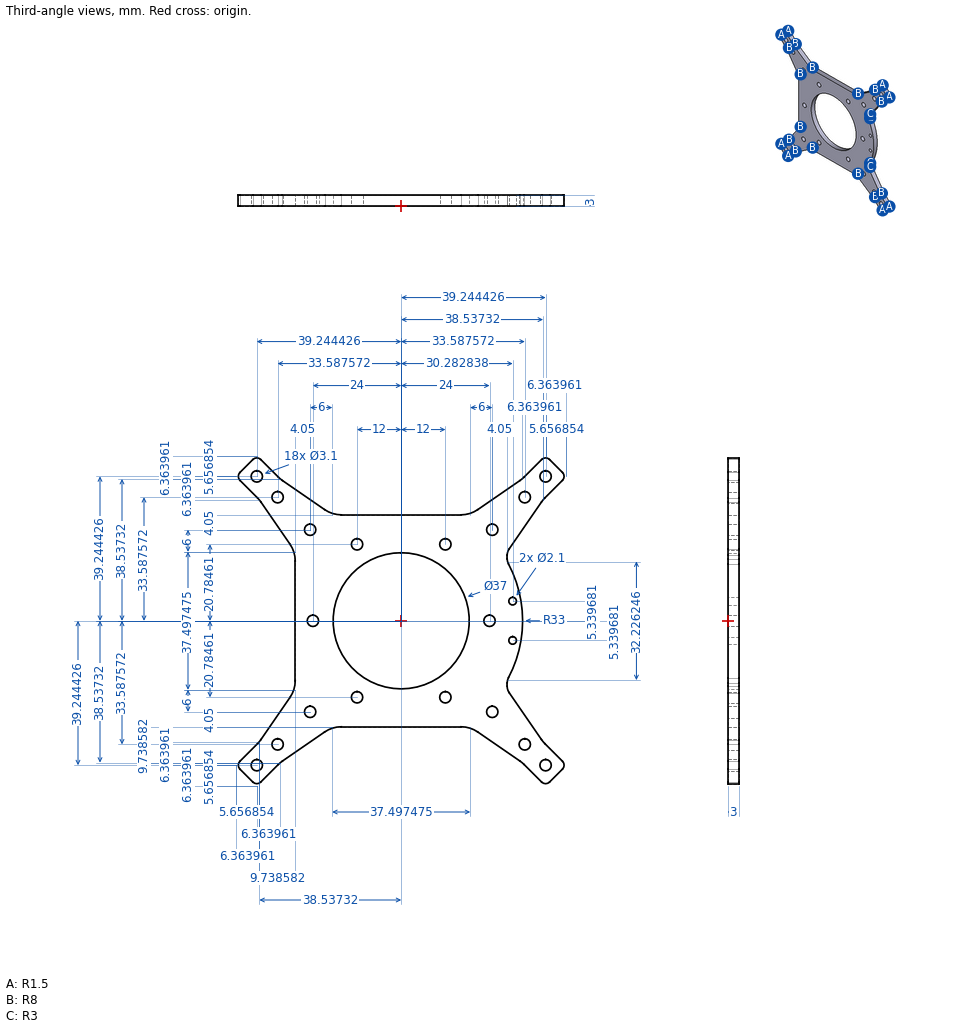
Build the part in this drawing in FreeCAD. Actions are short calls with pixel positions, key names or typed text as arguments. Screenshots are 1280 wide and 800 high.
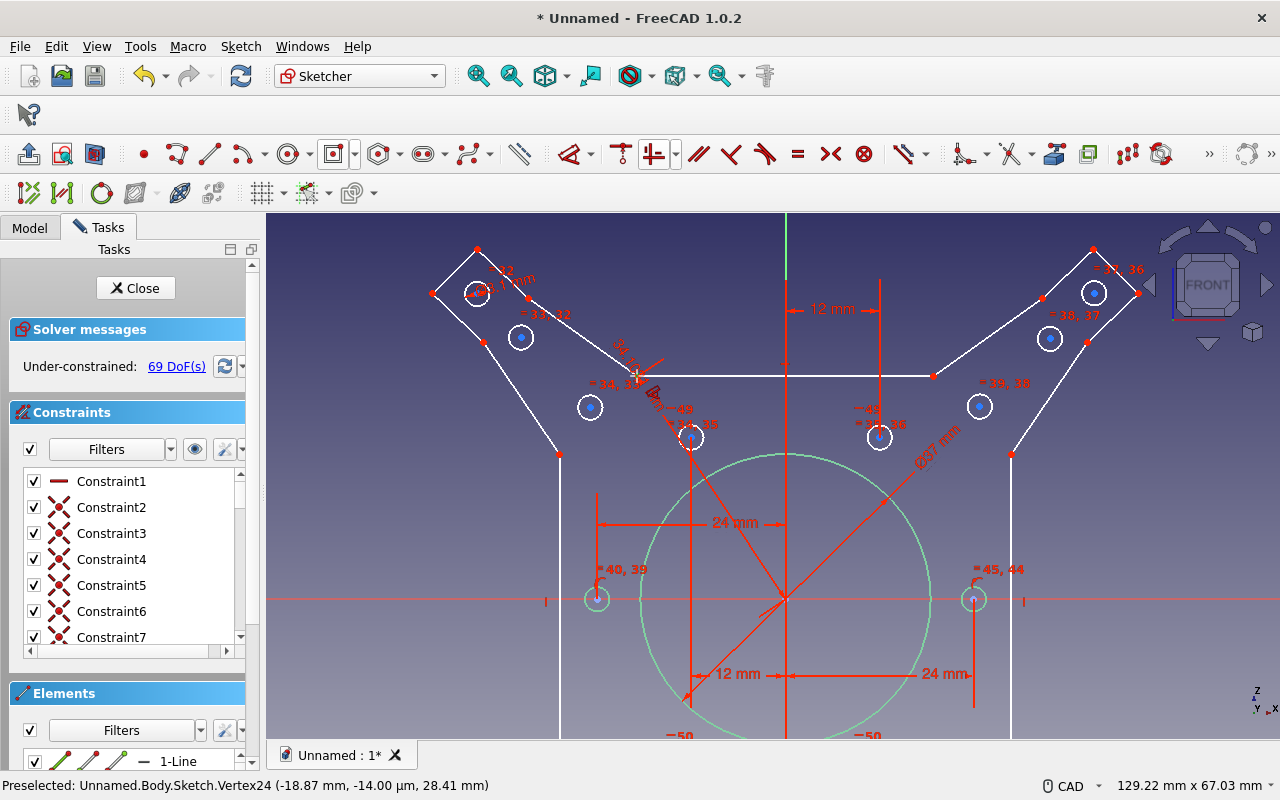
click(590, 408)
click(614, 342)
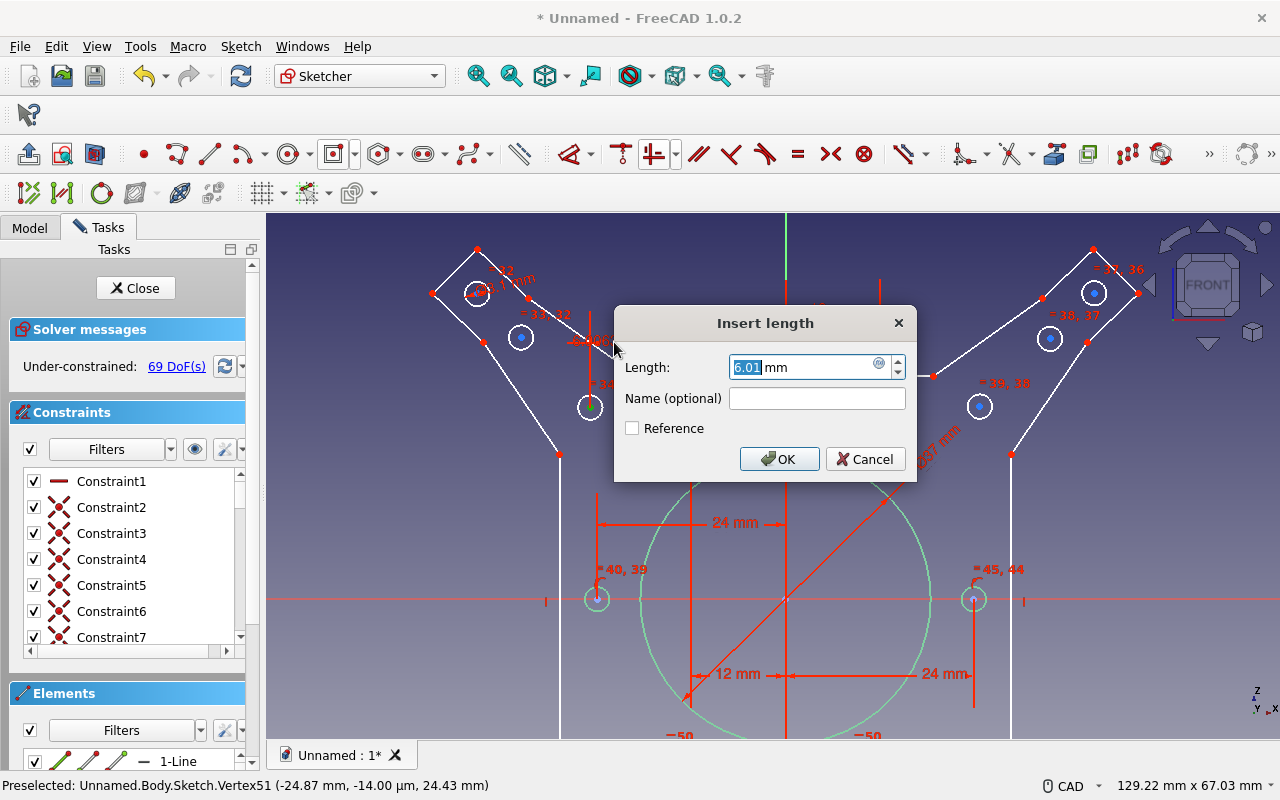
text(6)
key(Return)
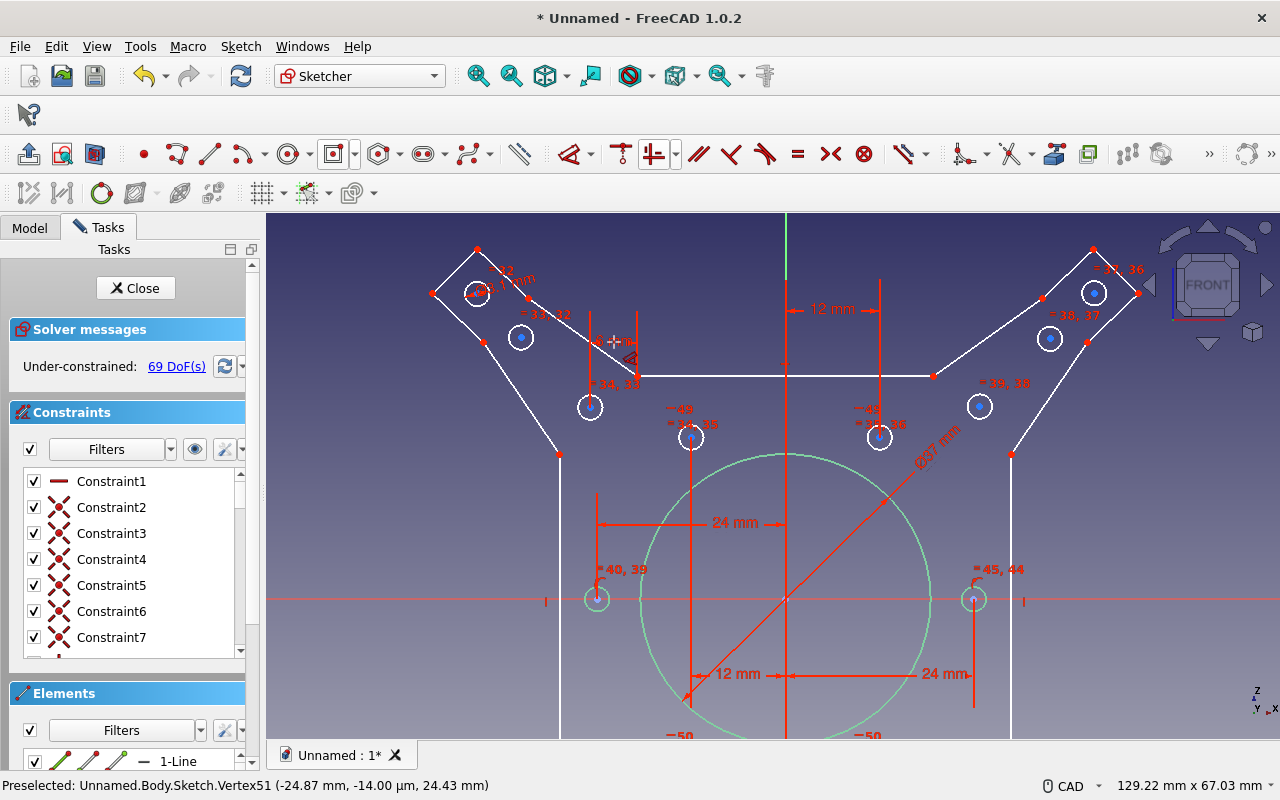
click(560, 454)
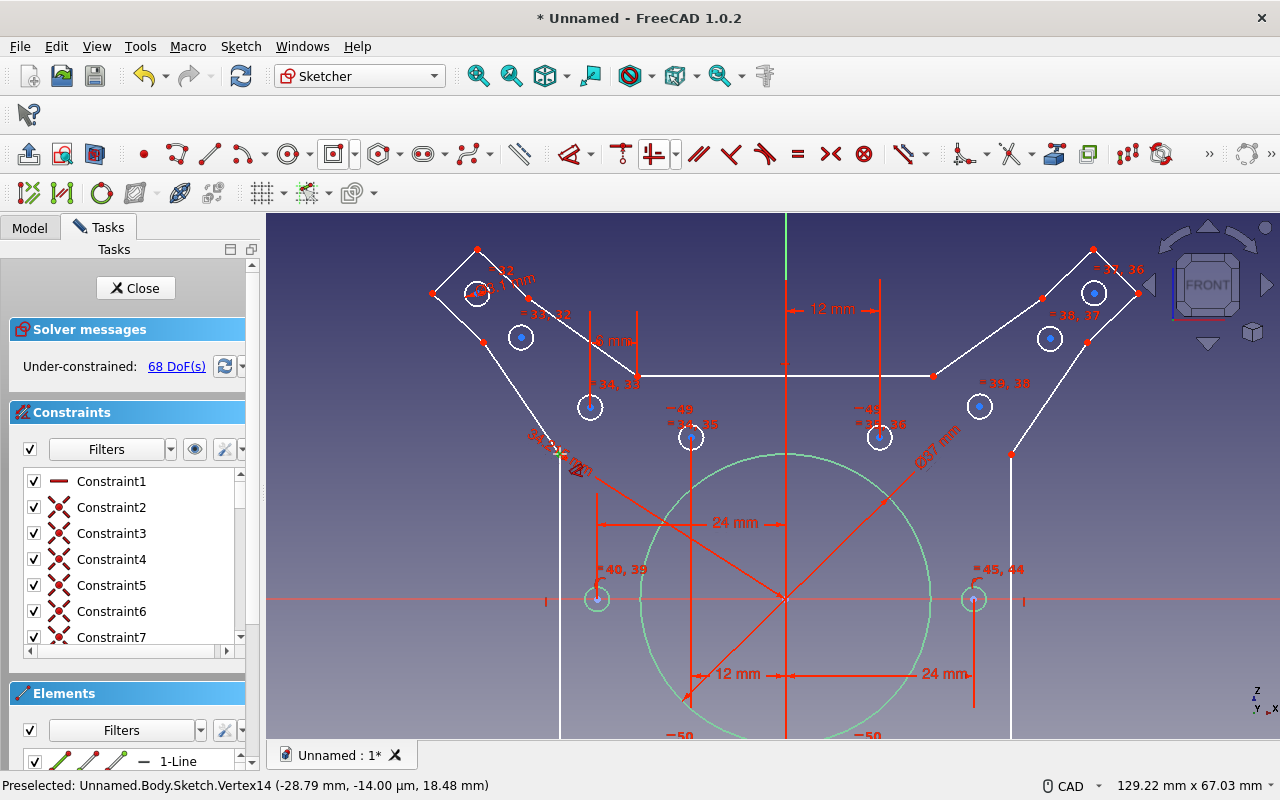
click(590, 408)
click(526, 431)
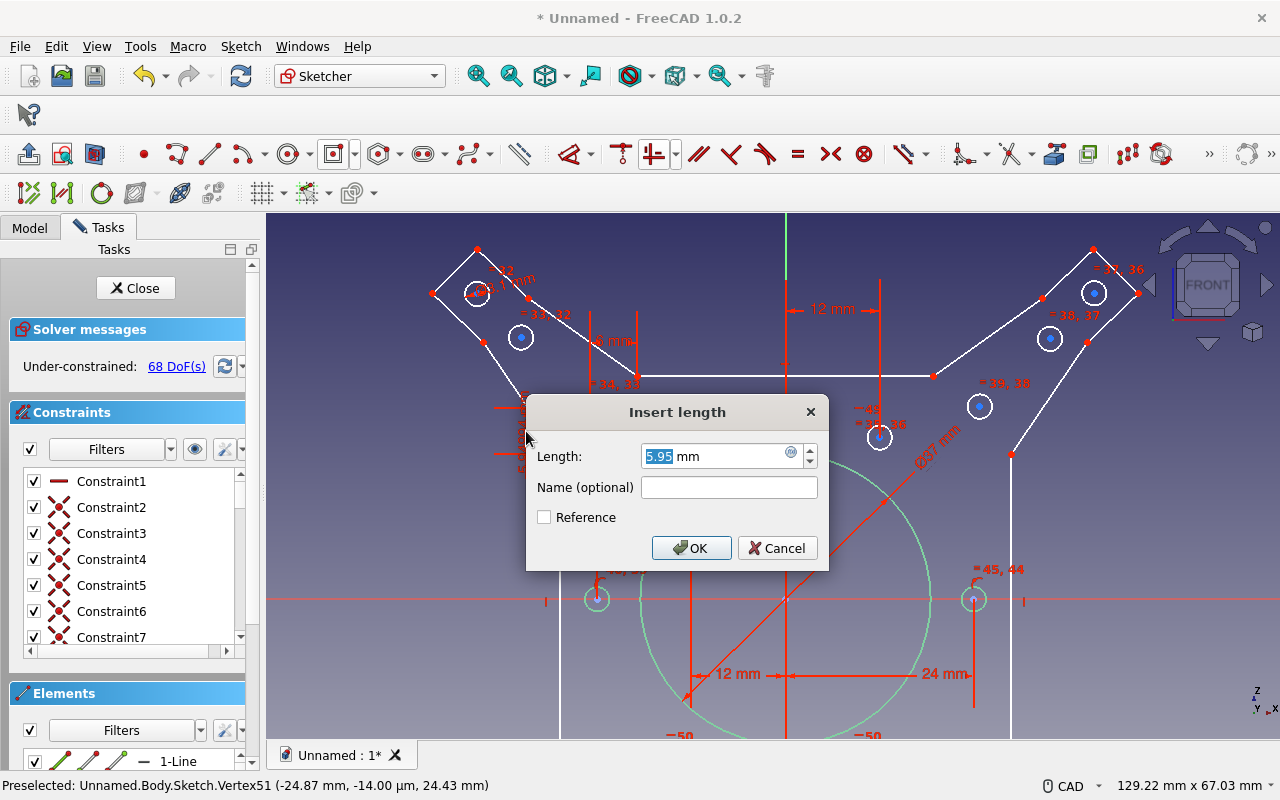
text(6)
key(Return)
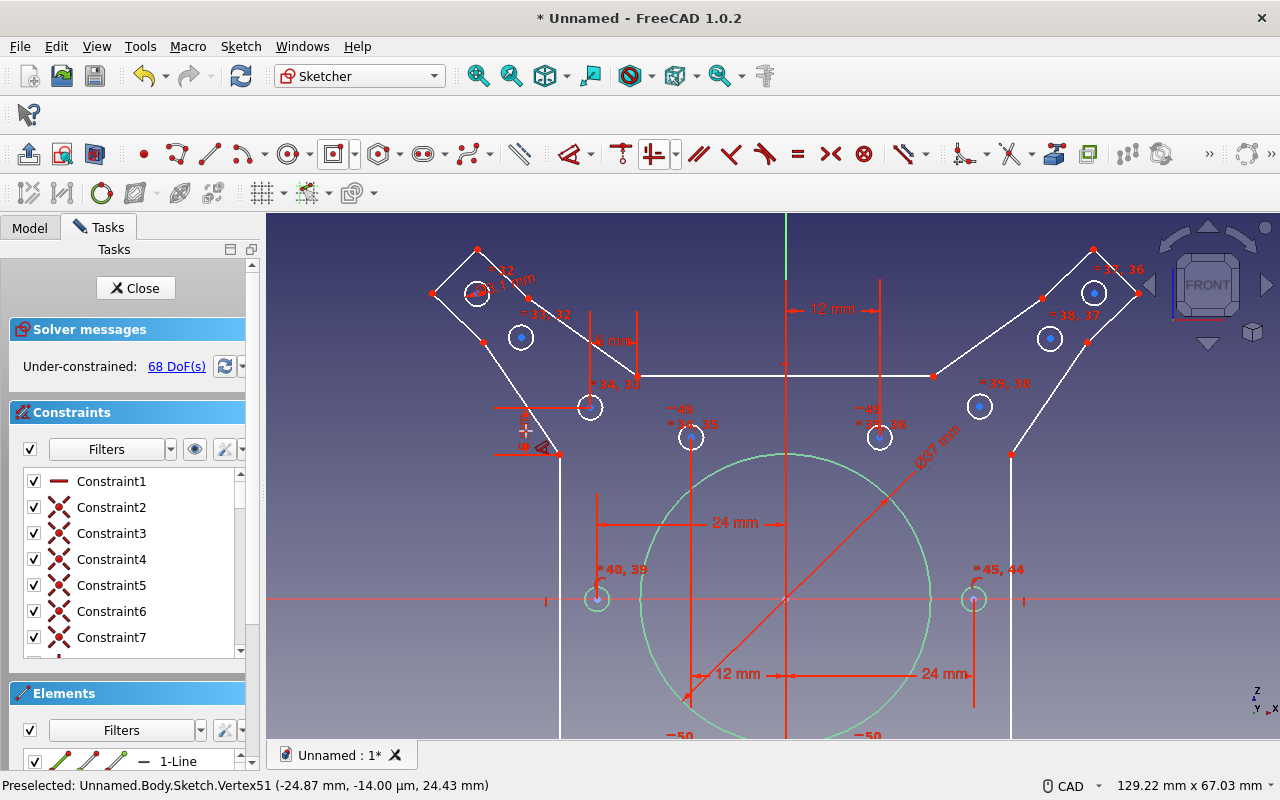
click(933, 376)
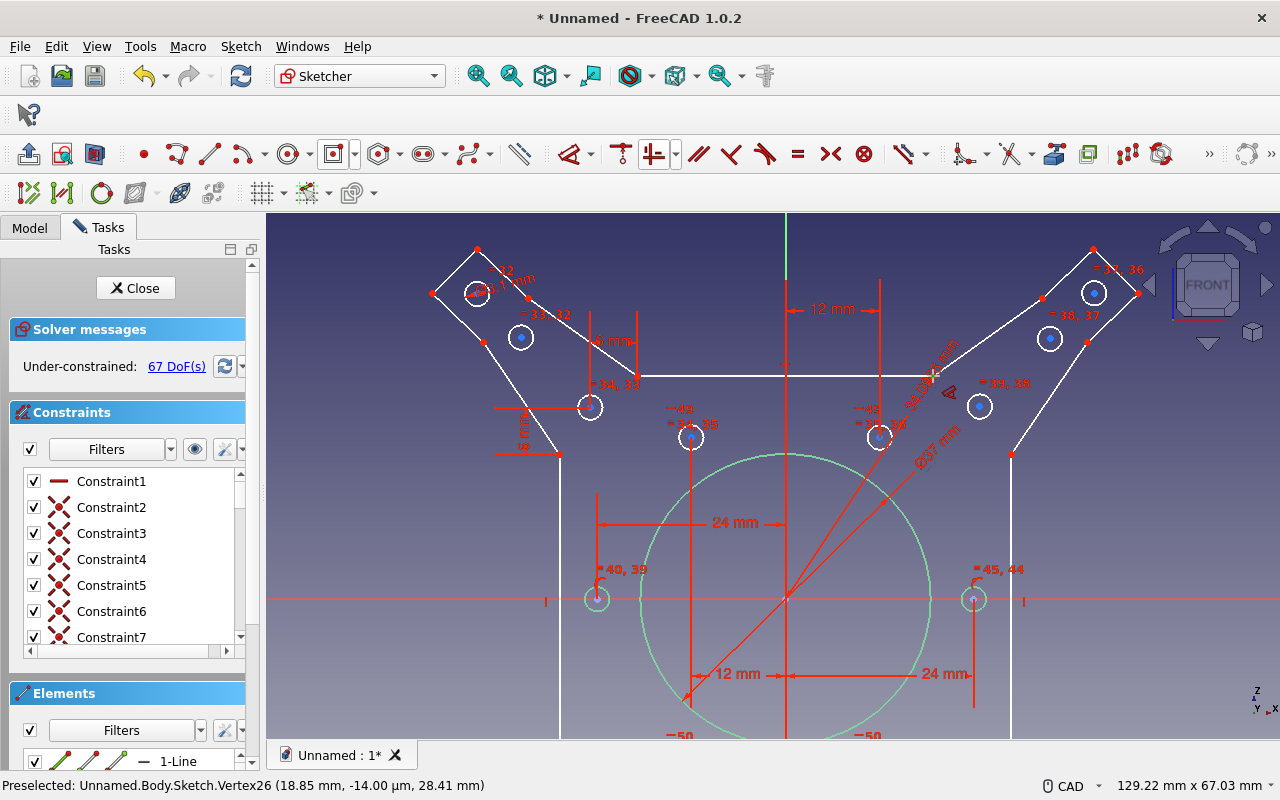
click(980, 407)
click(957, 342)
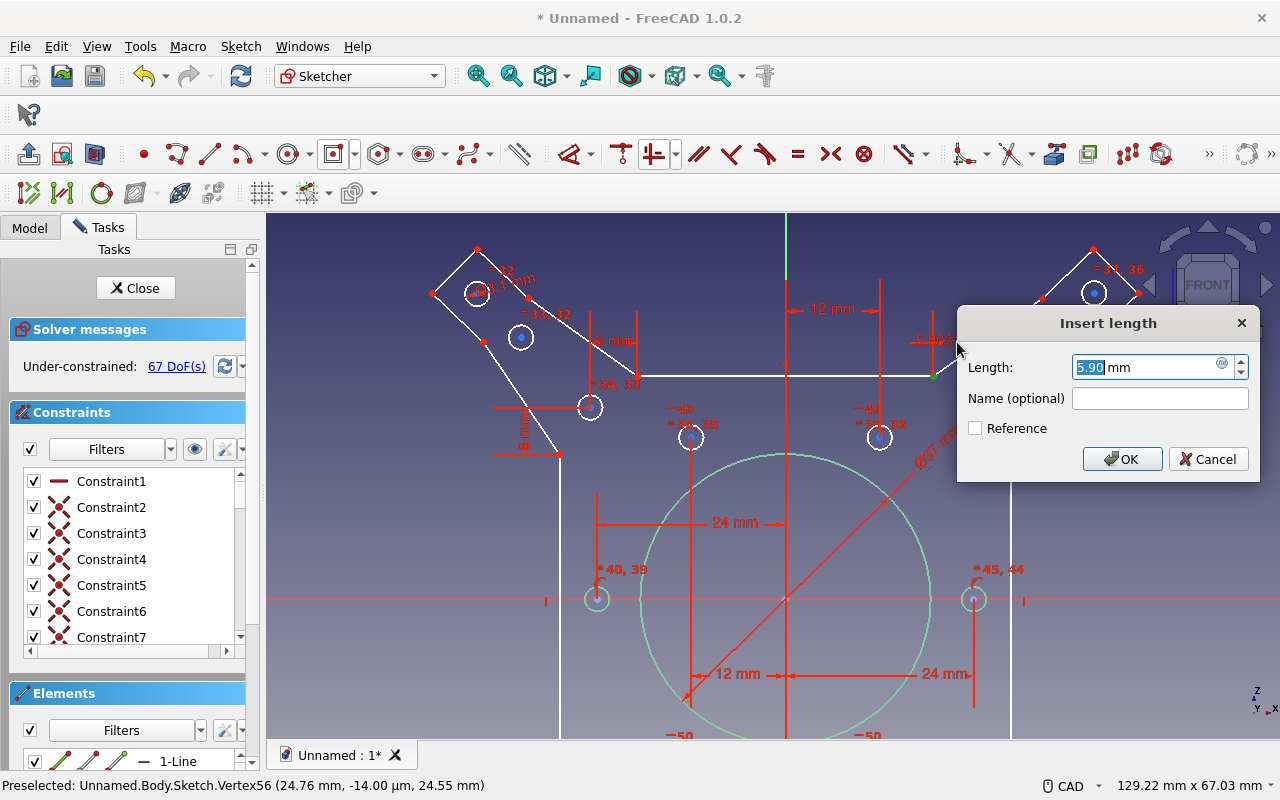
text(6)
key(Return)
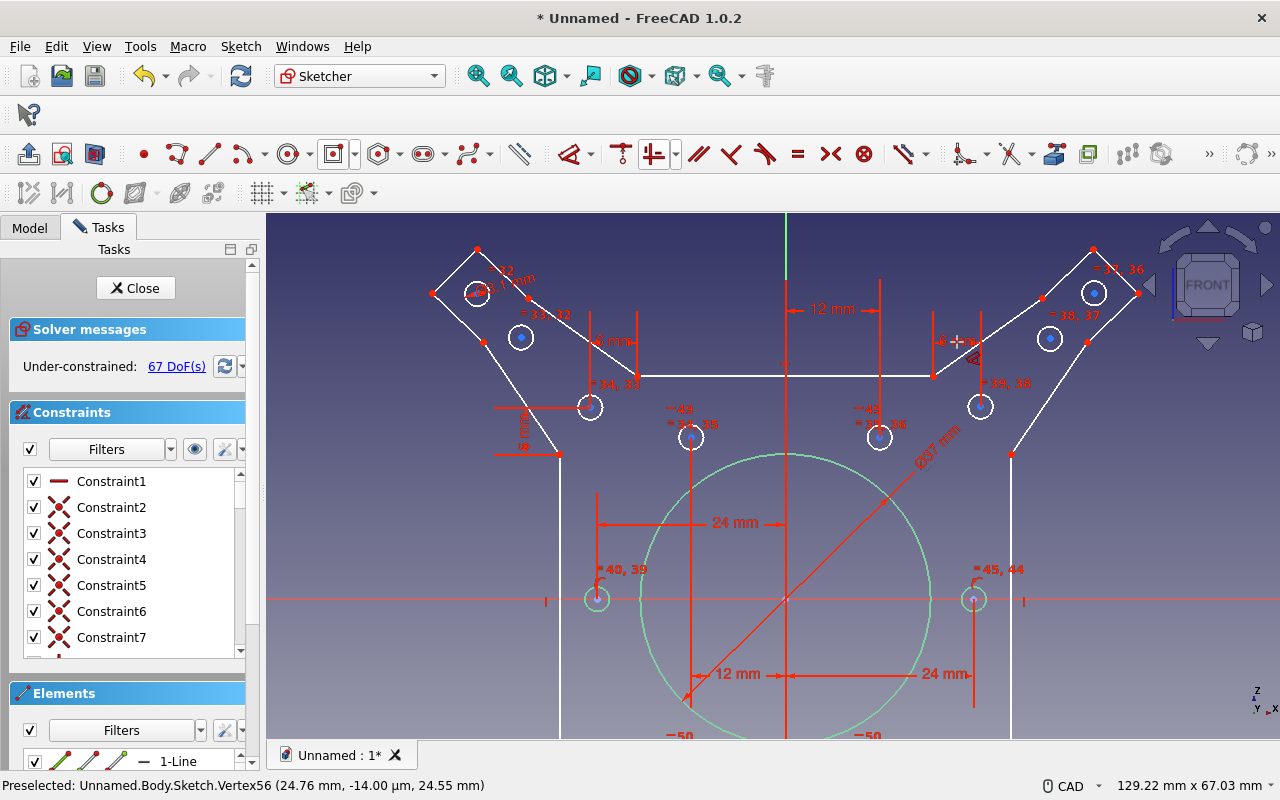
click(1011, 454)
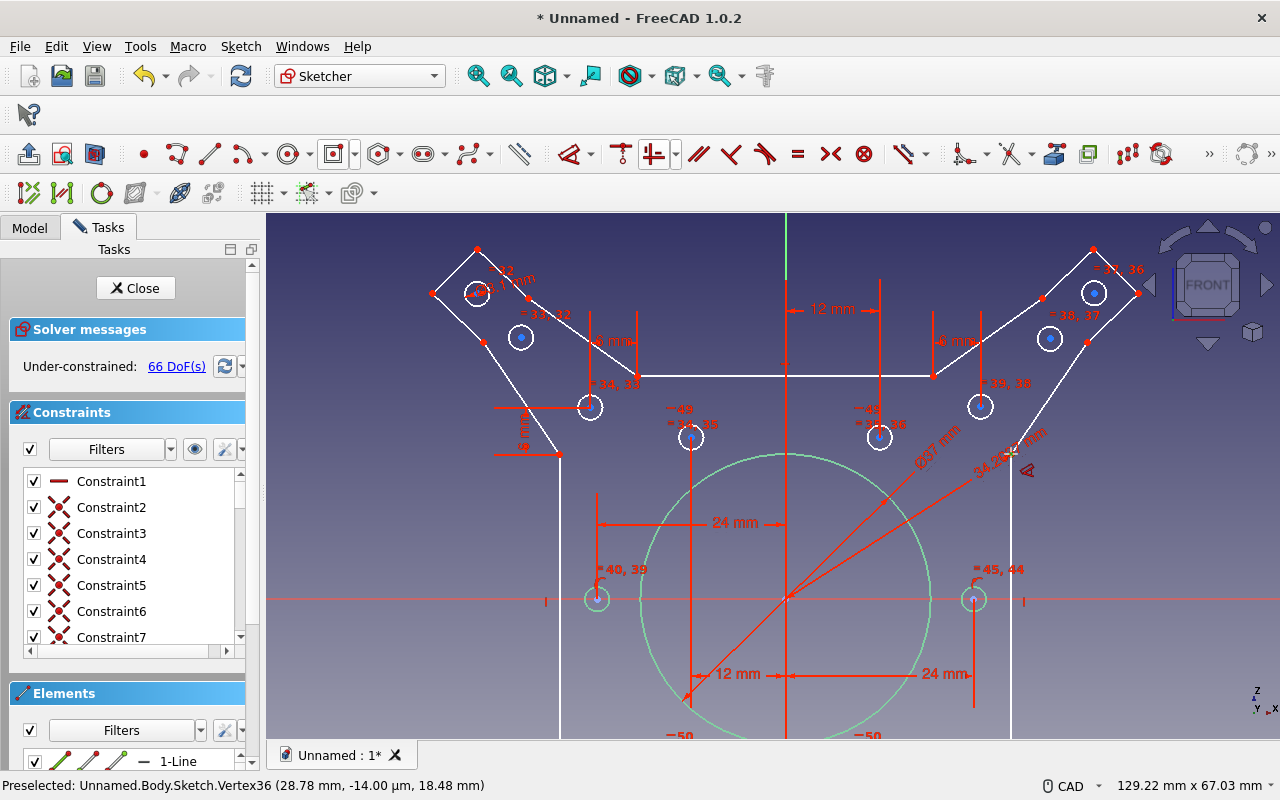
click(981, 407)
click(1045, 430)